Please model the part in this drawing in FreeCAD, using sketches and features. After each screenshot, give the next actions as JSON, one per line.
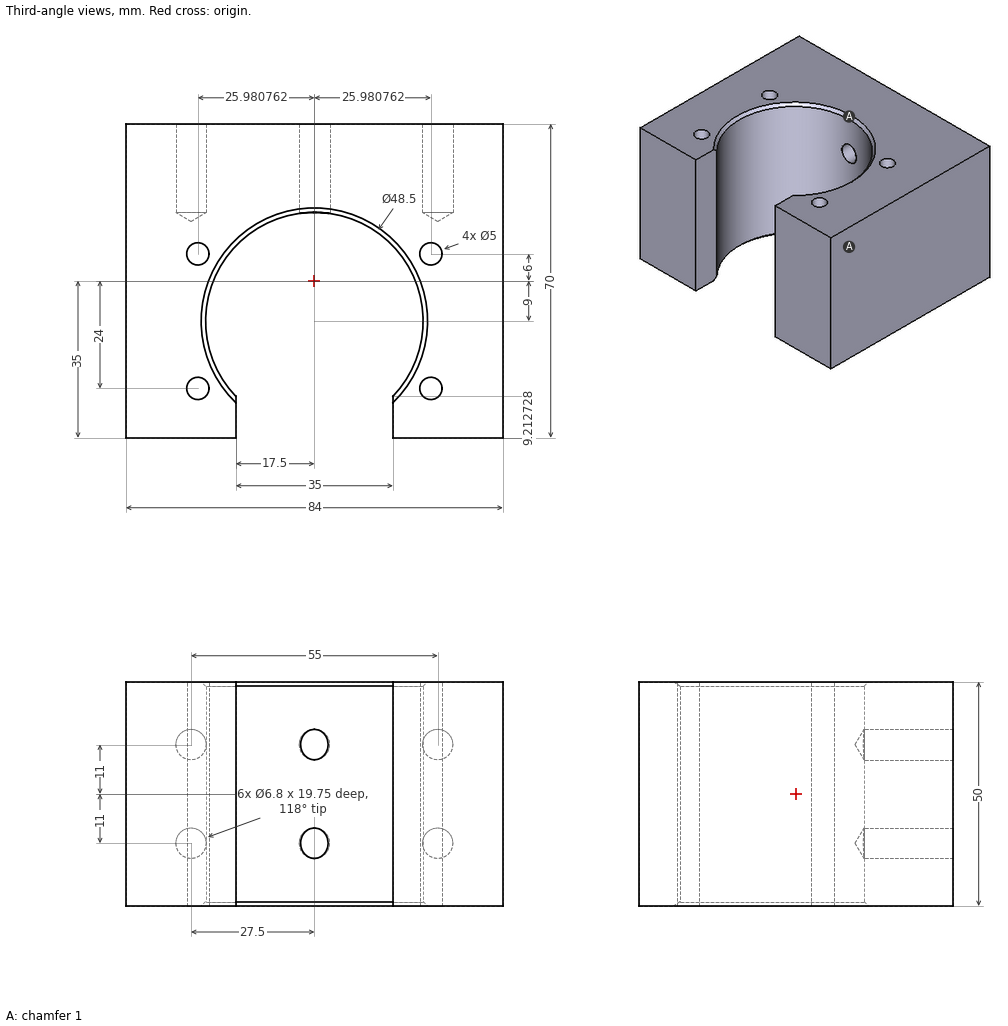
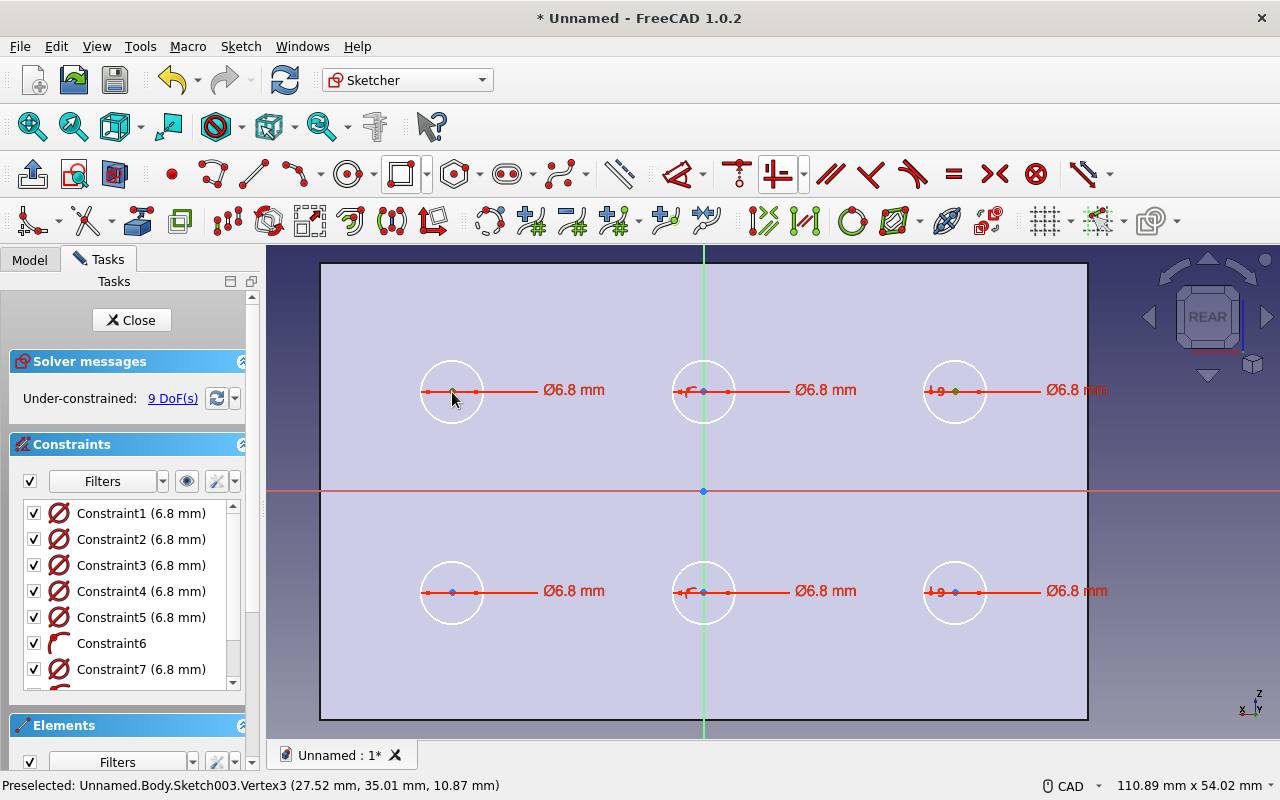
{"action": "key", "text": "h"}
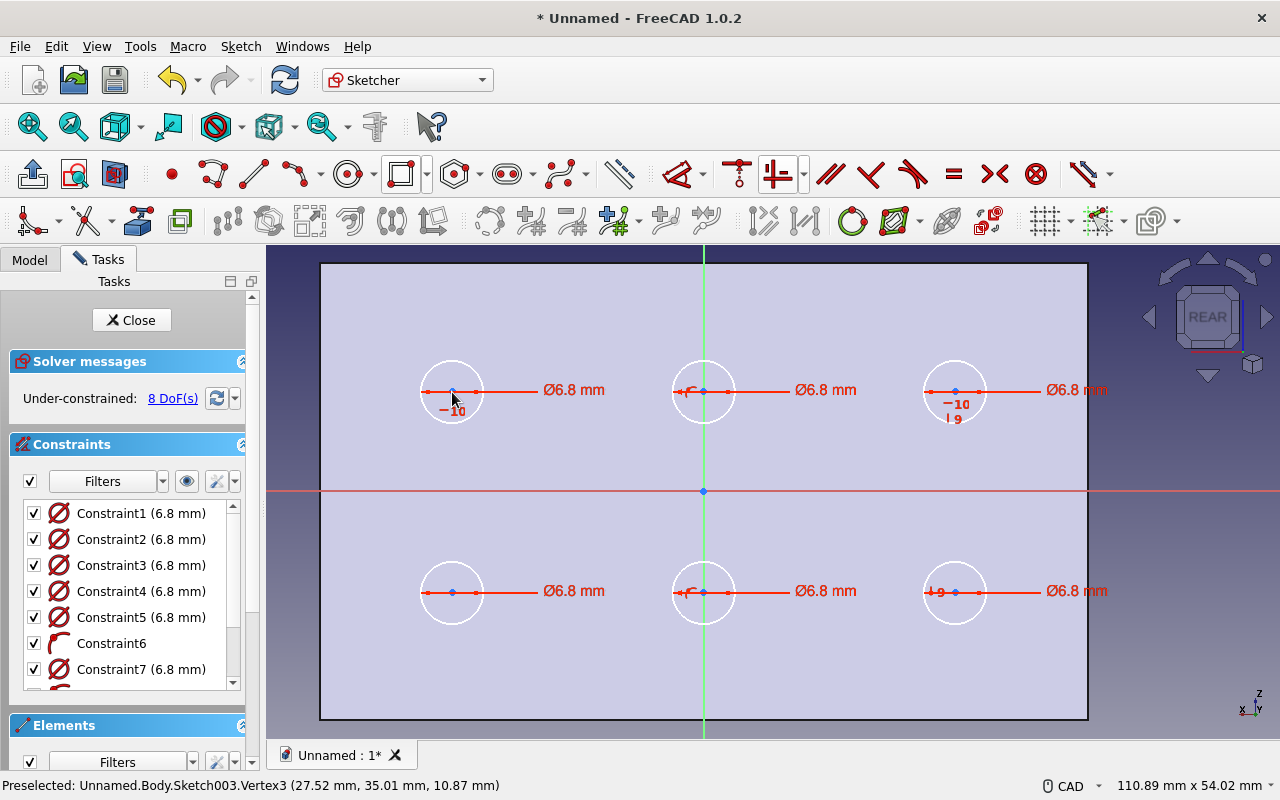
{"action": "left_click", "coordinate": [452, 392]}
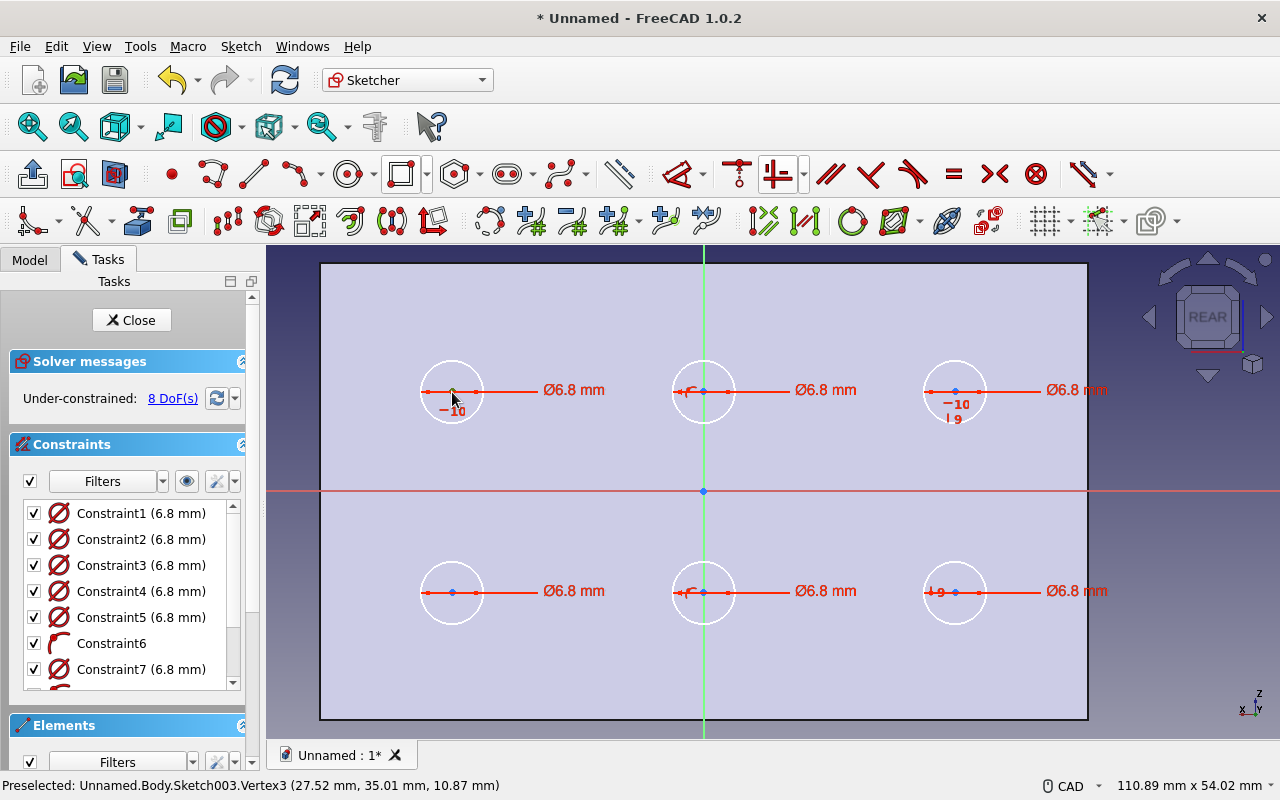
{"action": "left_click", "coordinate": [452, 593]}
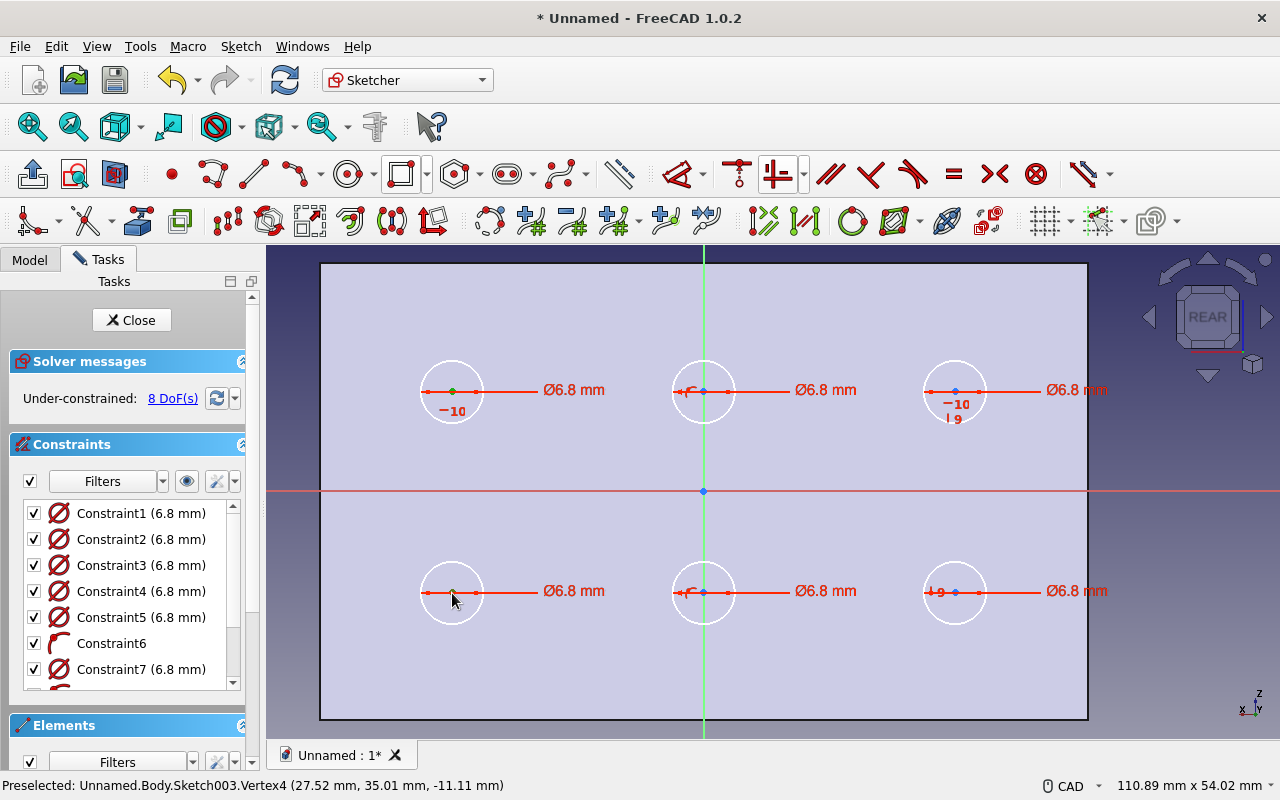
{"action": "left_click", "coordinate": [804, 174]}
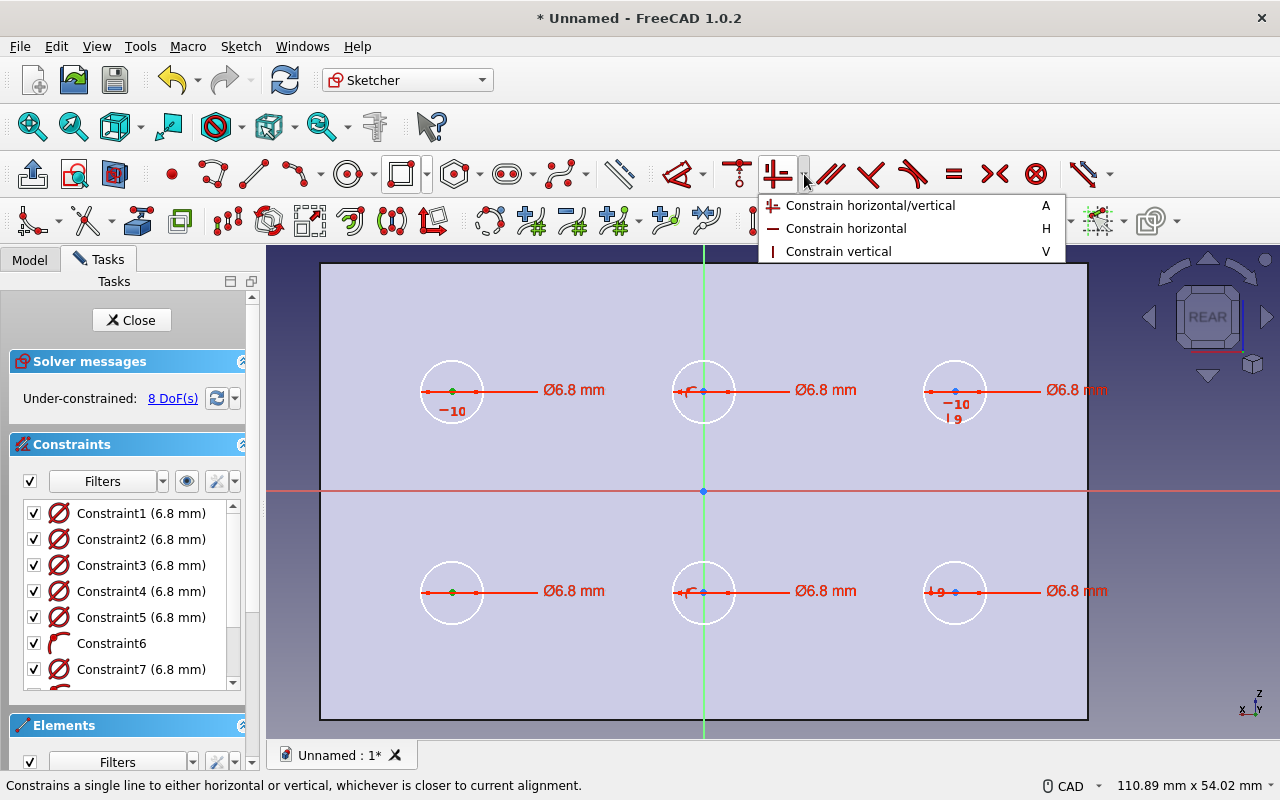
{"action": "left_click", "coordinate": [912, 252]}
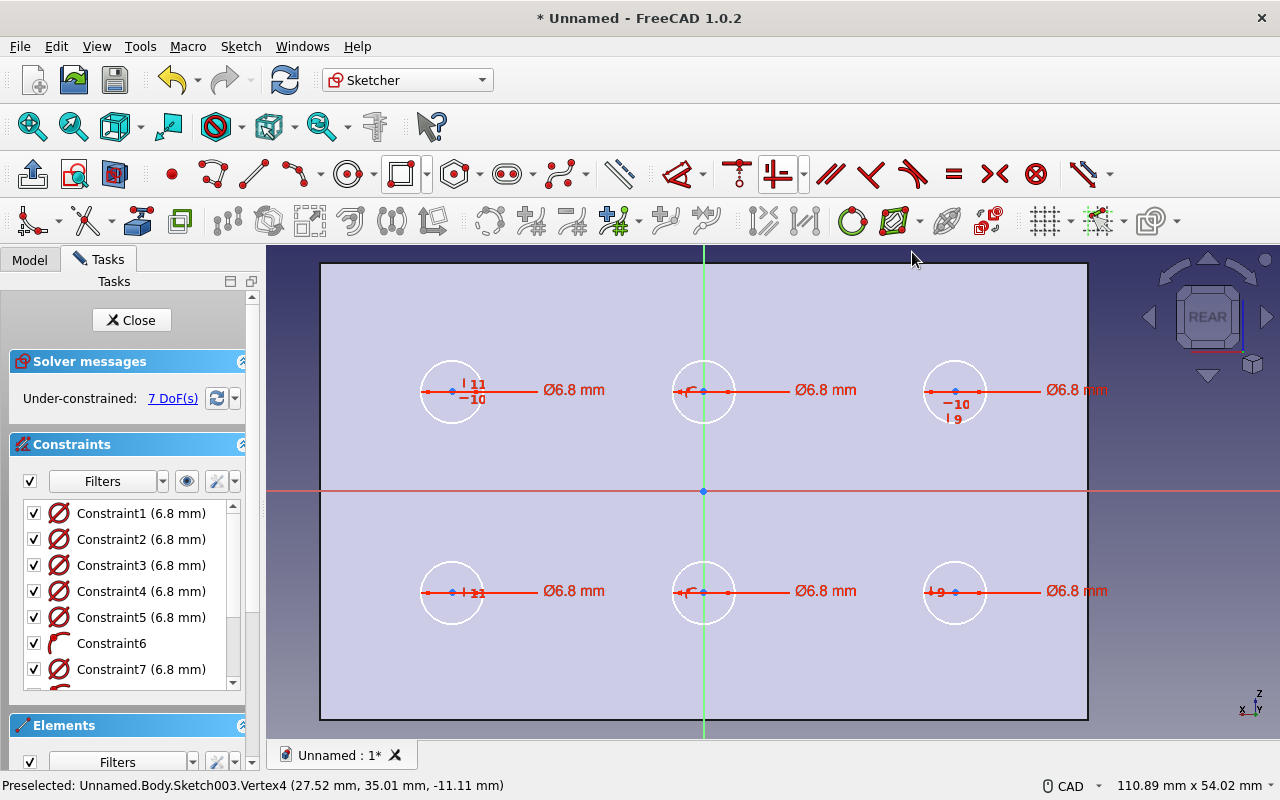
{"action": "left_click", "coordinate": [955, 593]}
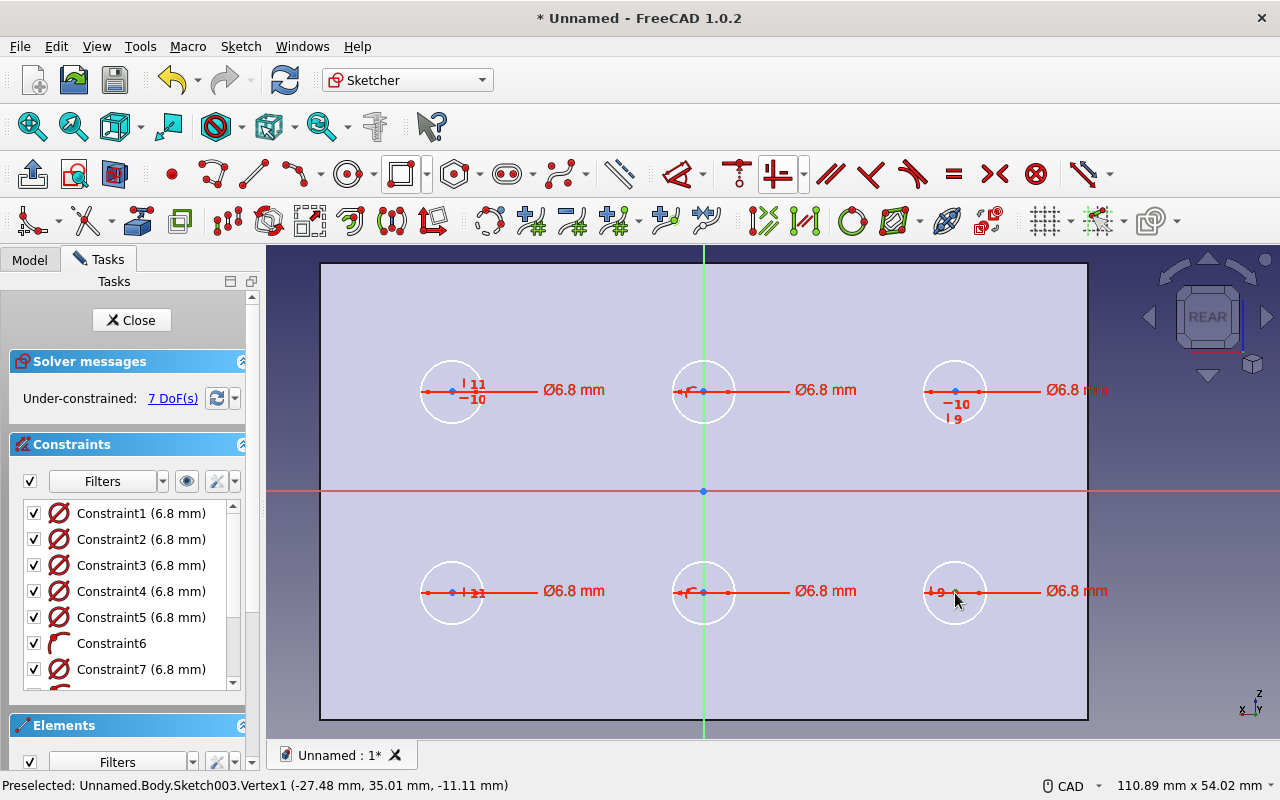
{"action": "left_click", "coordinate": [452, 593]}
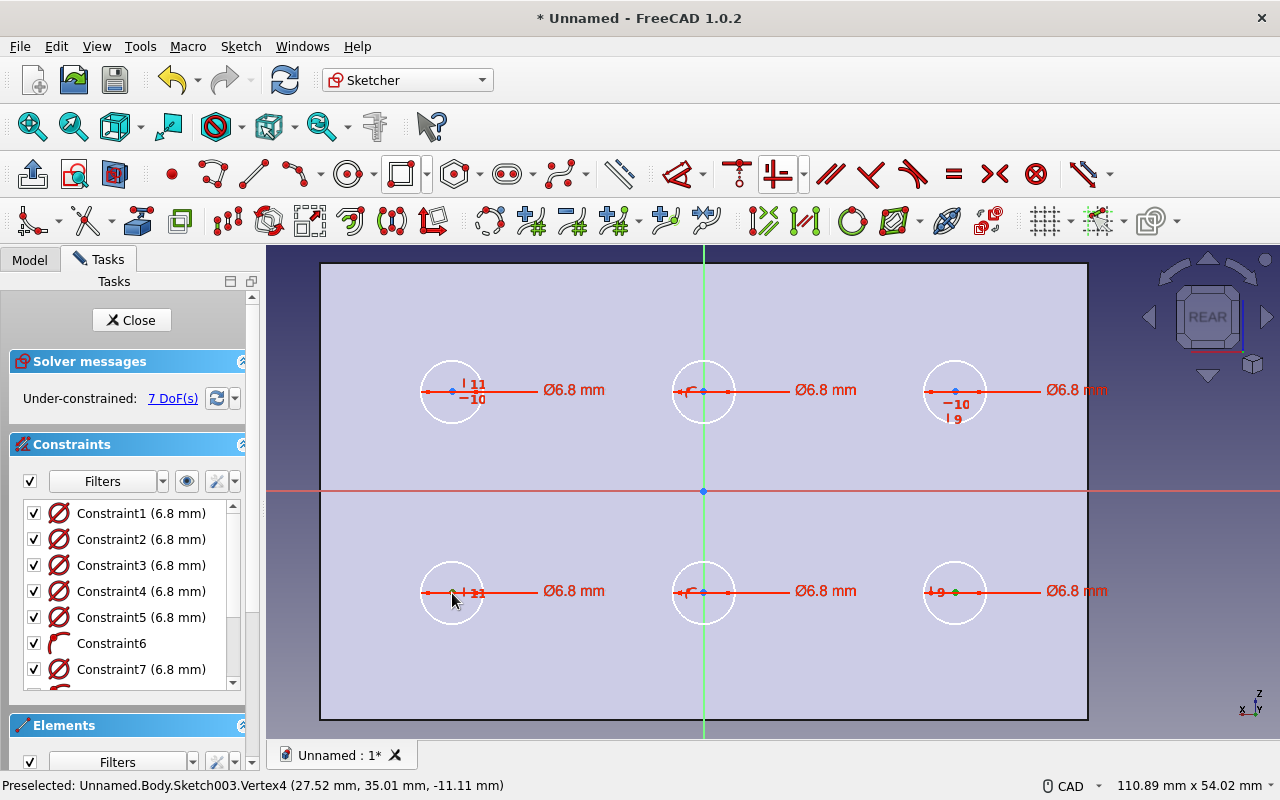
{"action": "left_click", "coordinate": [804, 174]}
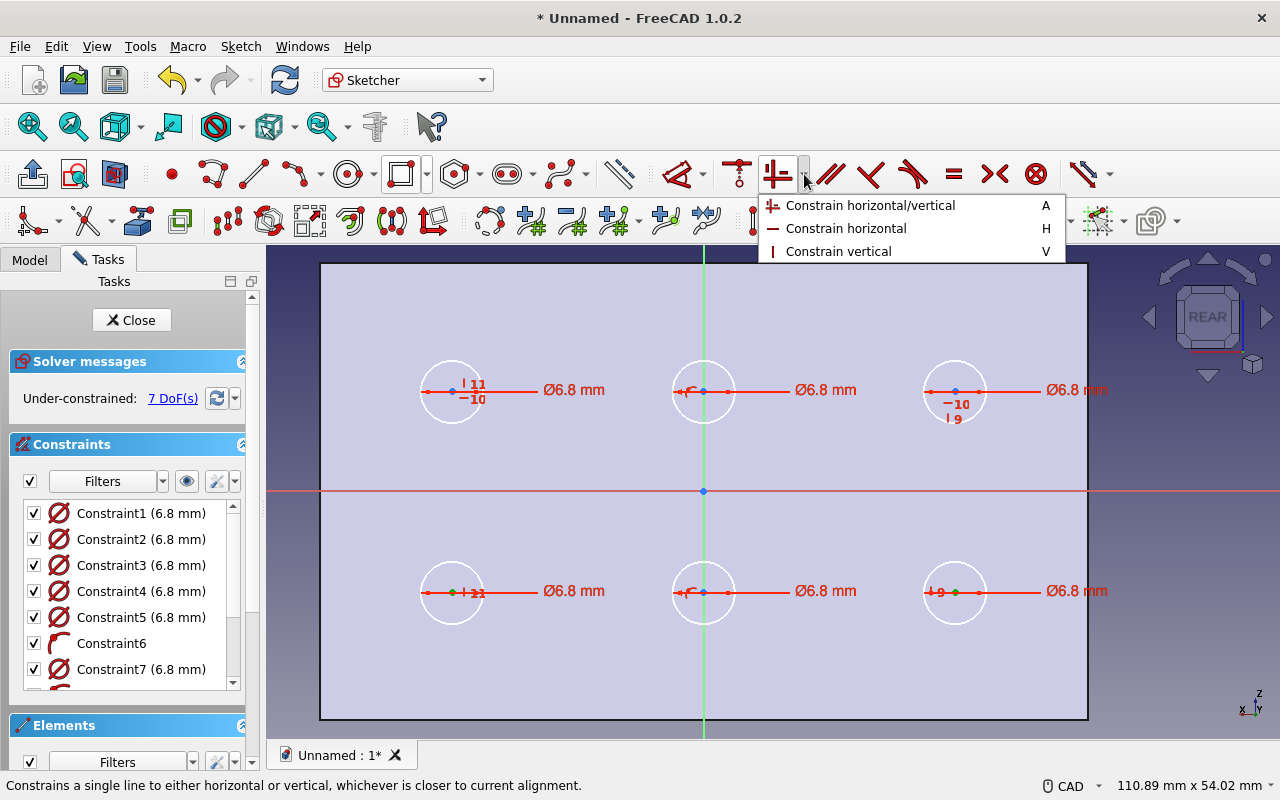
{"action": "left_click", "coordinate": [912, 228]}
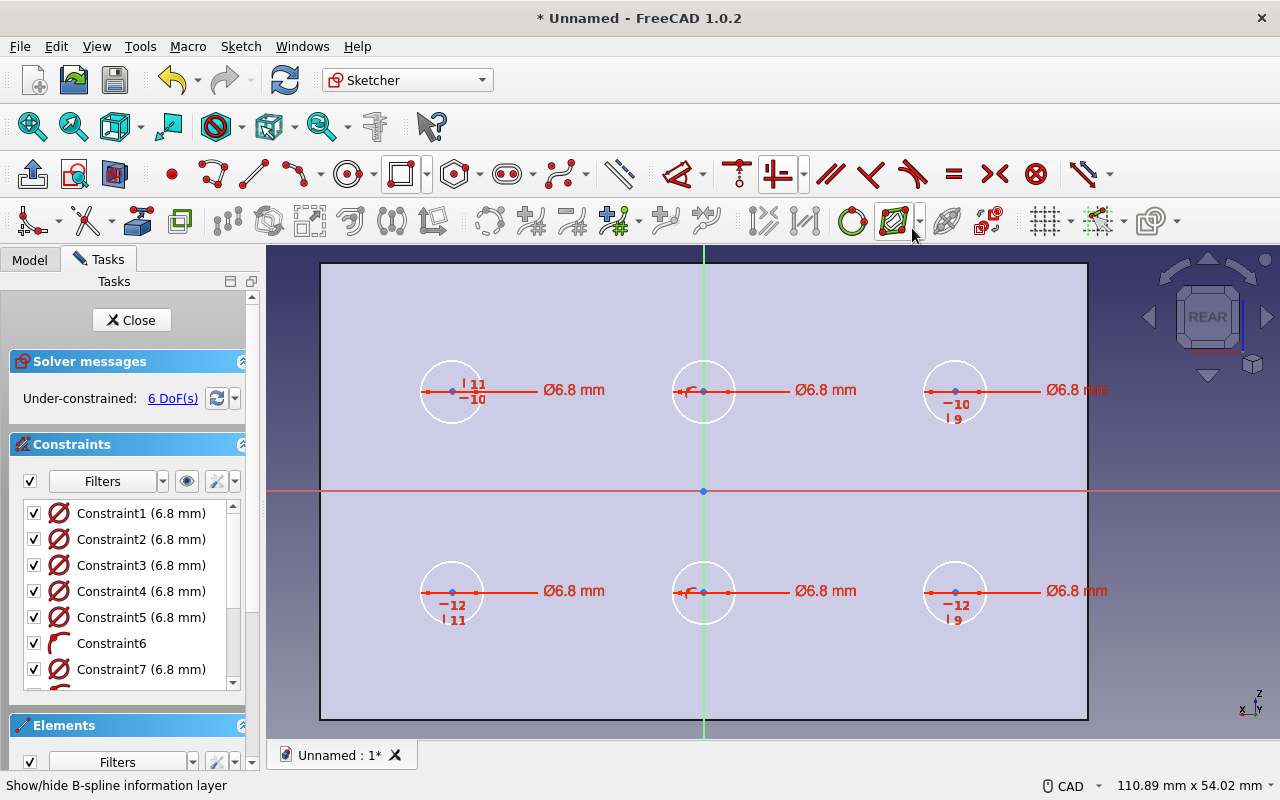
{"action": "left_click", "coordinate": [955, 593]}